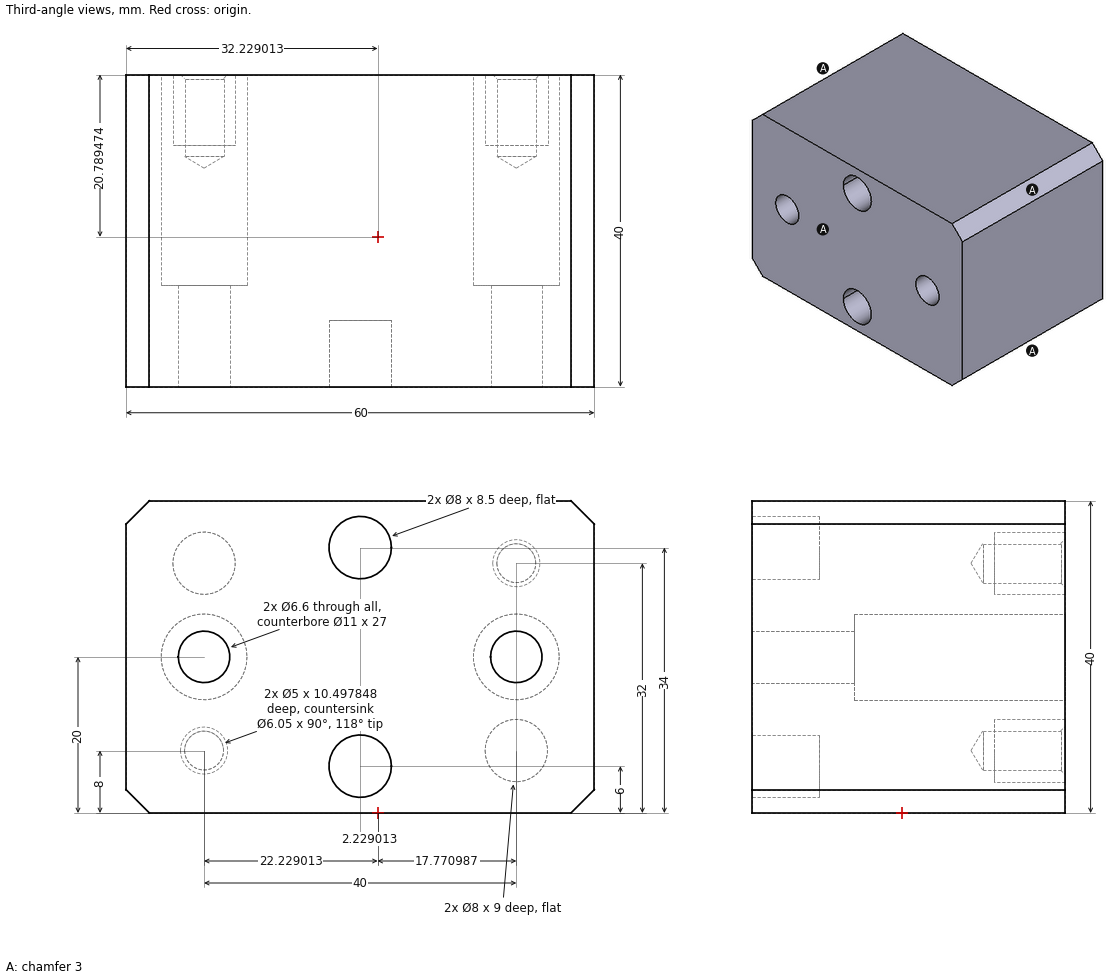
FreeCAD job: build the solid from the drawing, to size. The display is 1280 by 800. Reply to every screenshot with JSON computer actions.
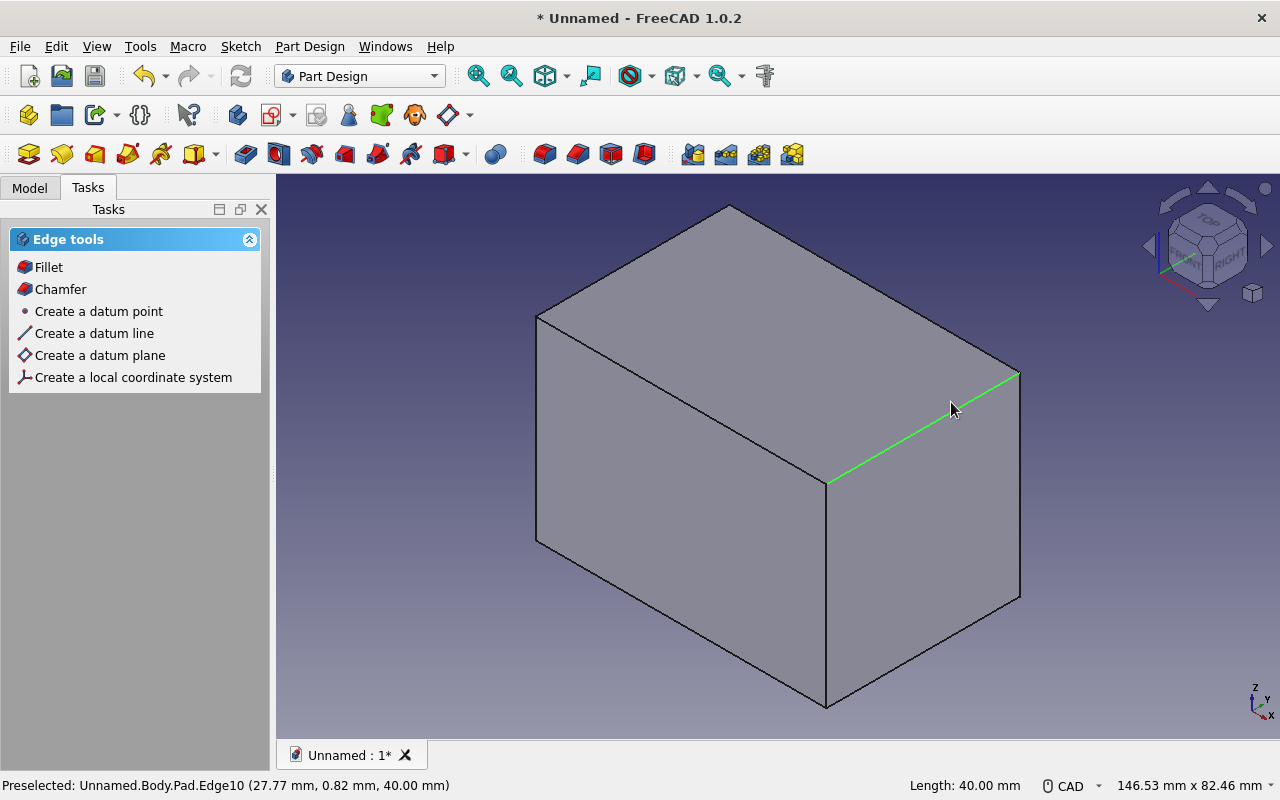
{"action": "key", "text": "2"}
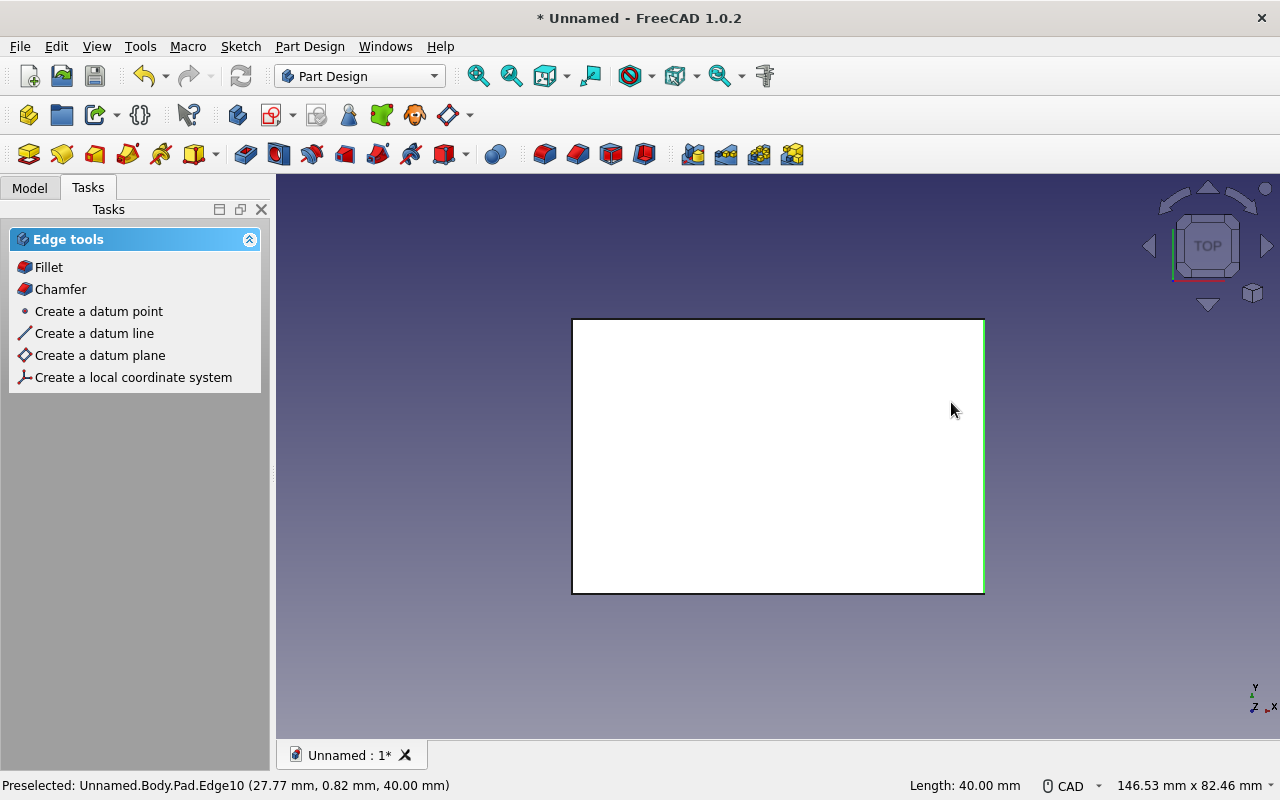
{"action": "left_click", "coordinate": [572, 456], "text": "ctrl"}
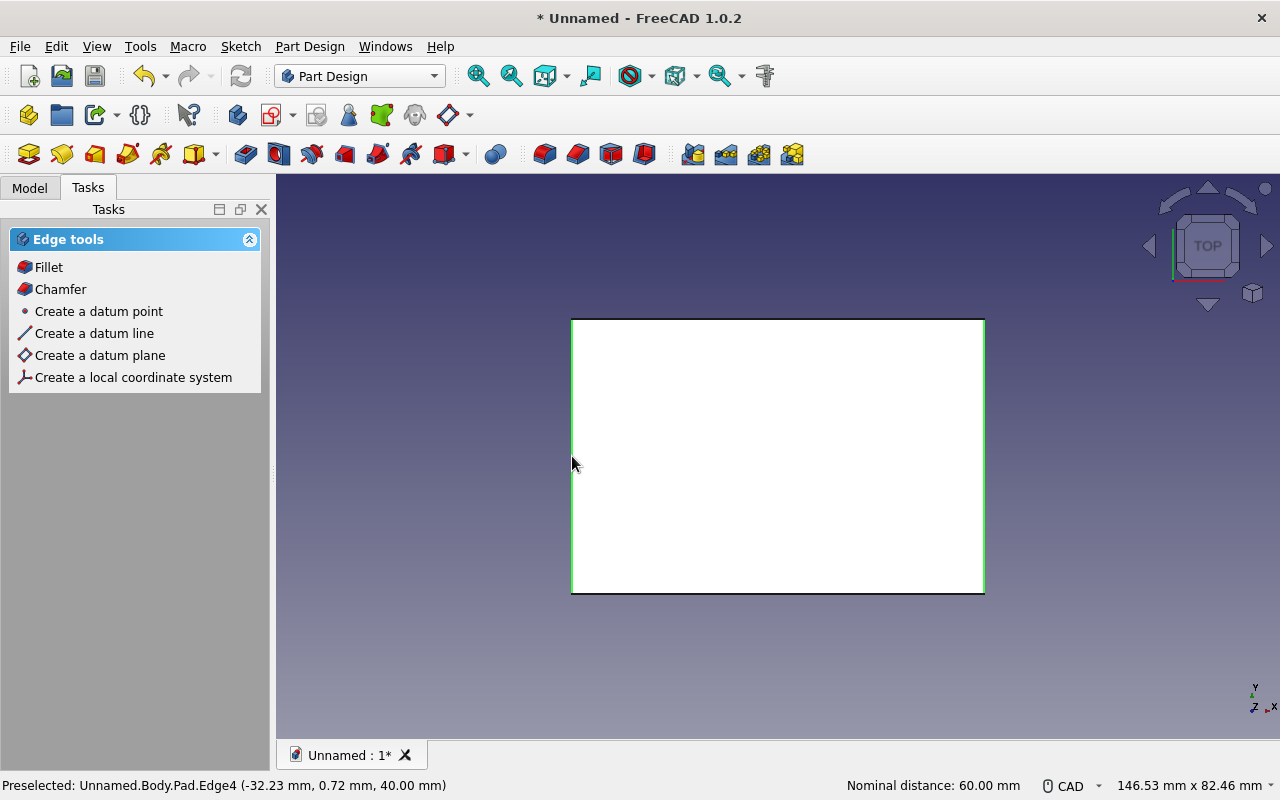
{"action": "key", "text": "1"}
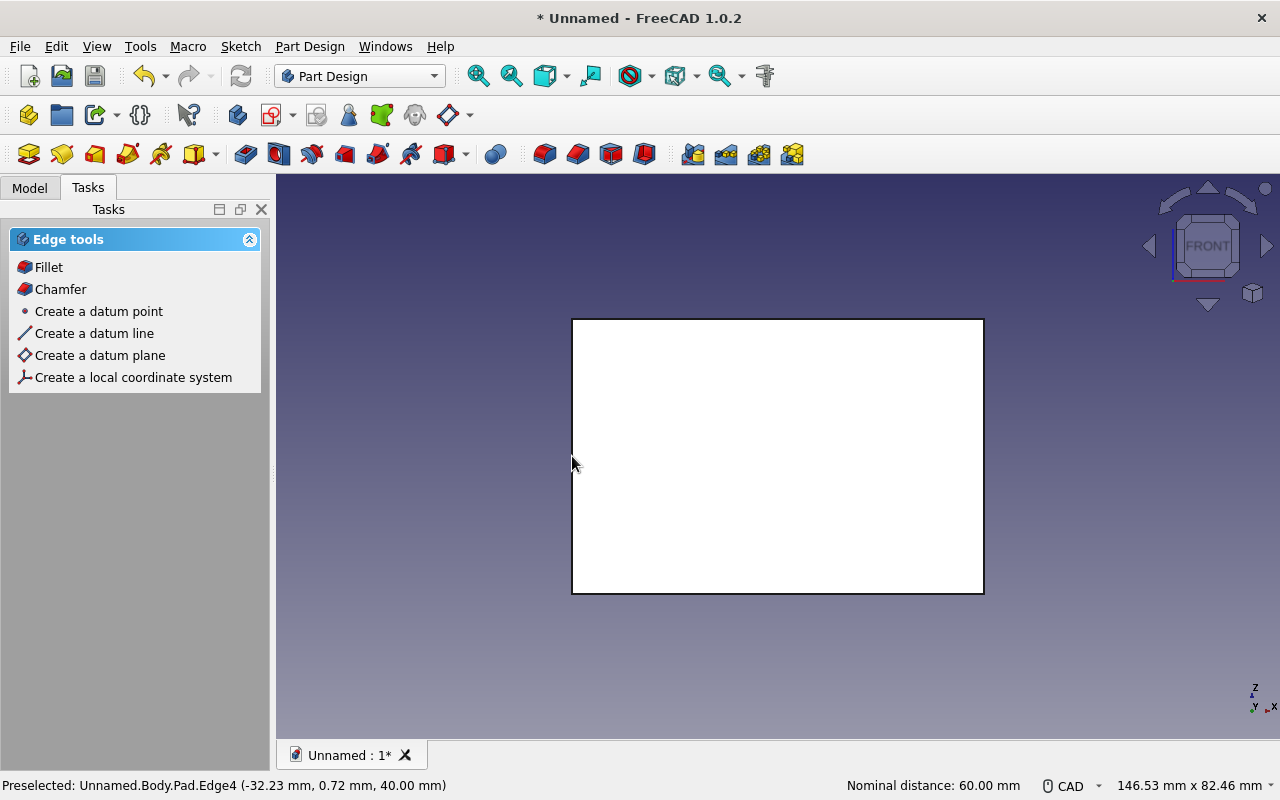
{"action": "key", "text": "3"}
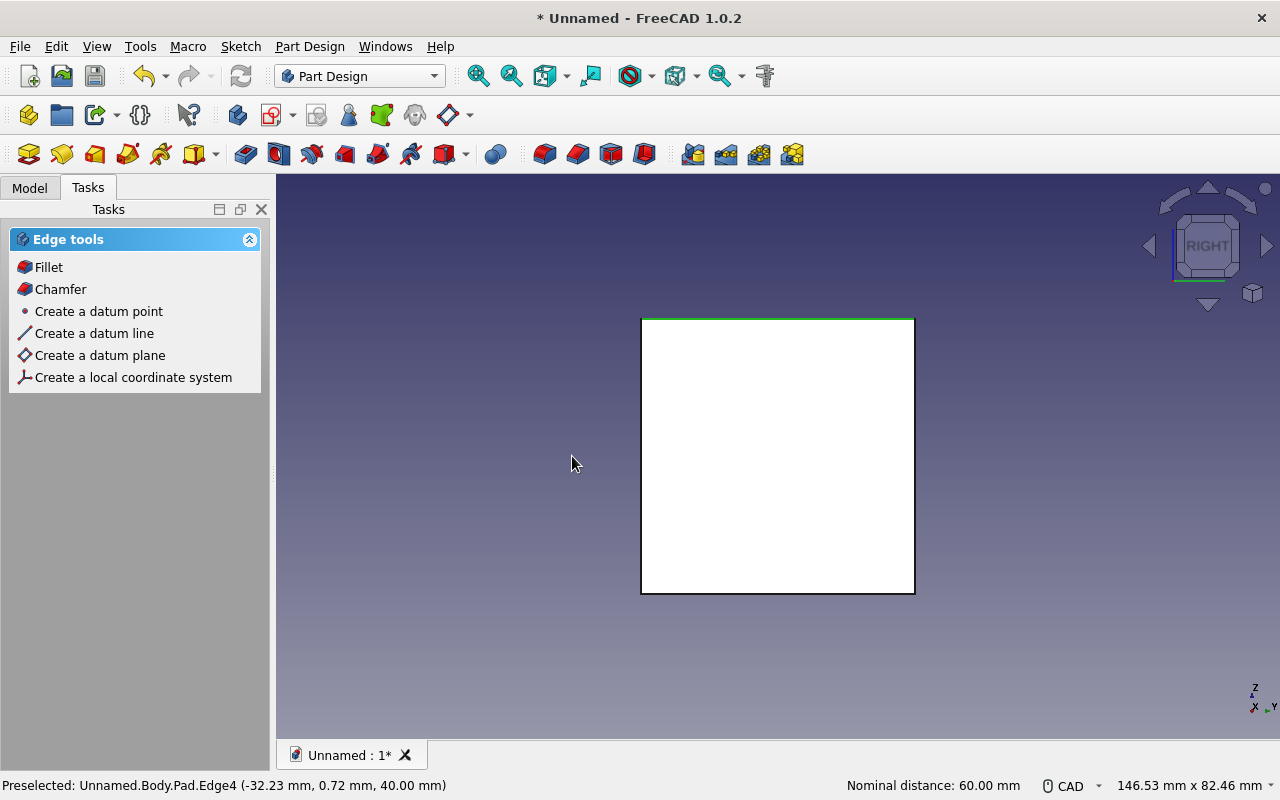
{"action": "left_click", "coordinate": [778, 593], "text": "ctrl"}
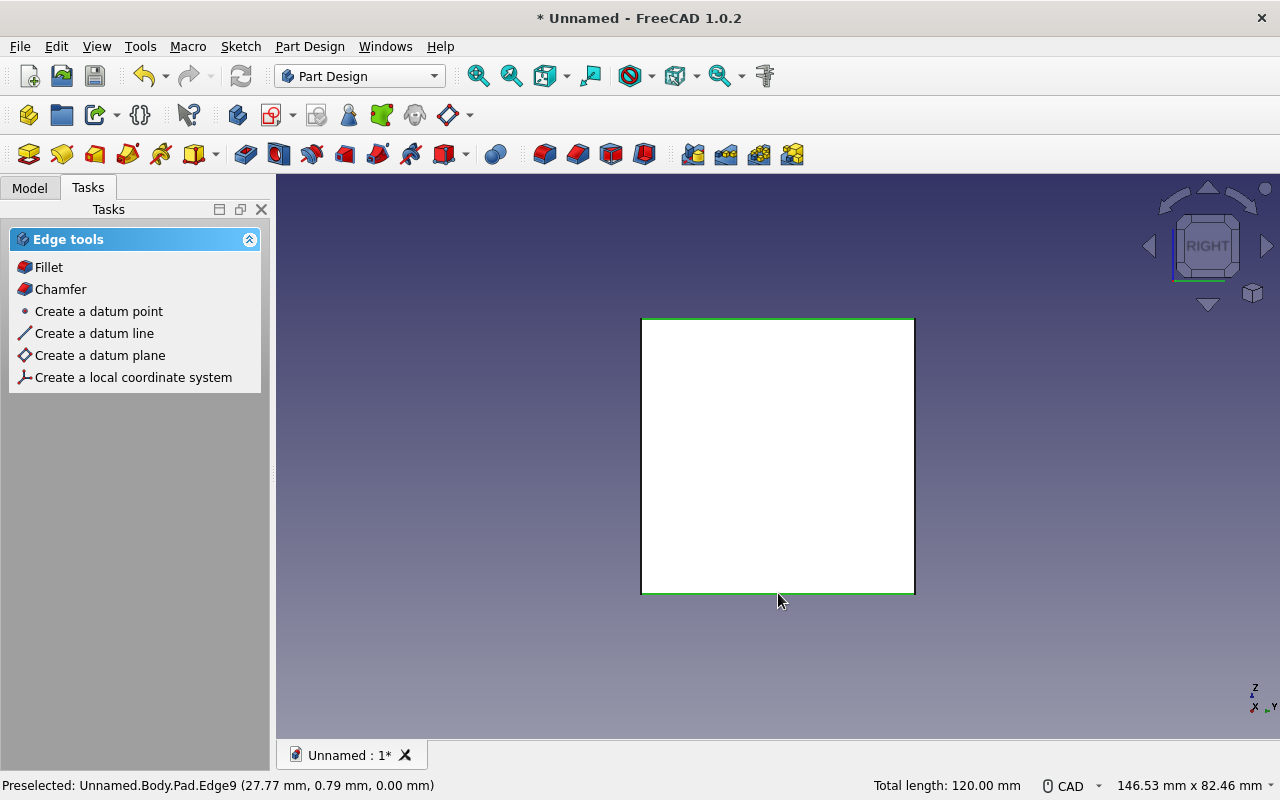
{"action": "key", "text": "5"}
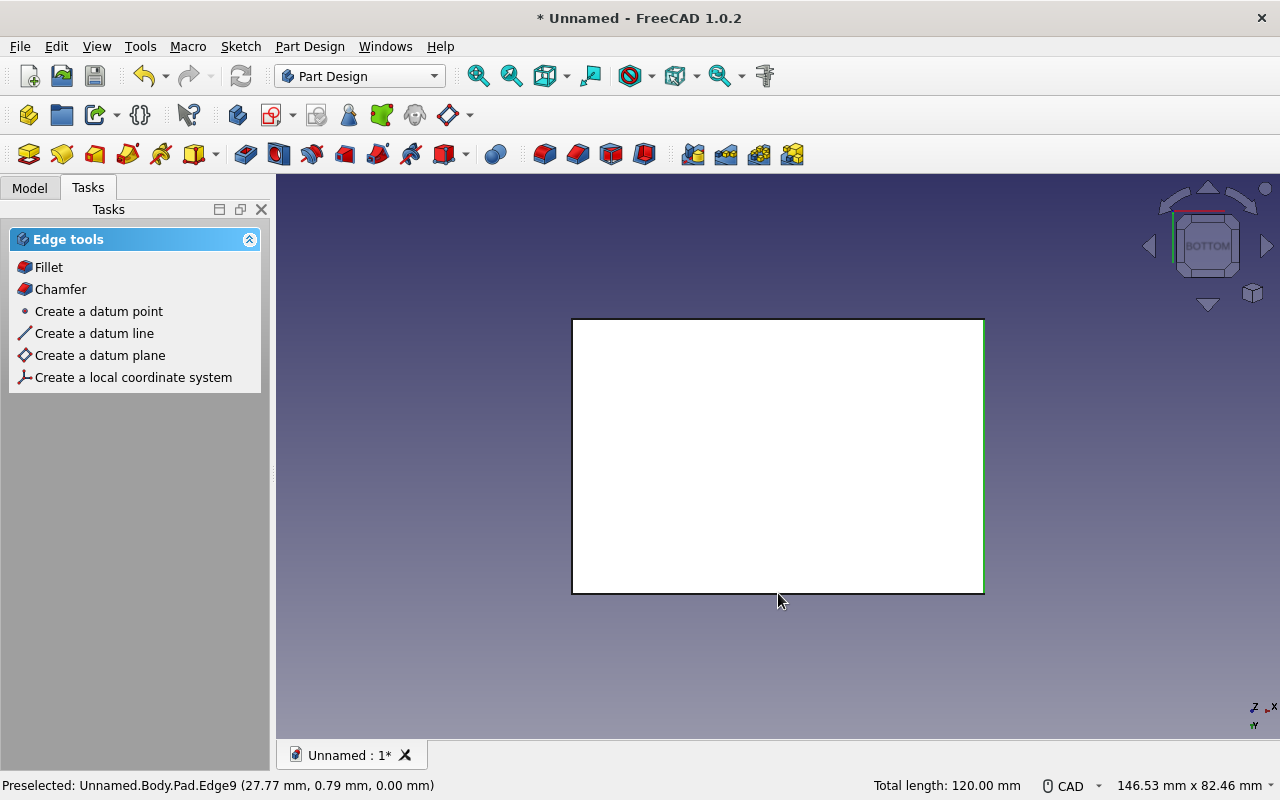
{"action": "left_click", "coordinate": [572, 455], "text": "ctrl"}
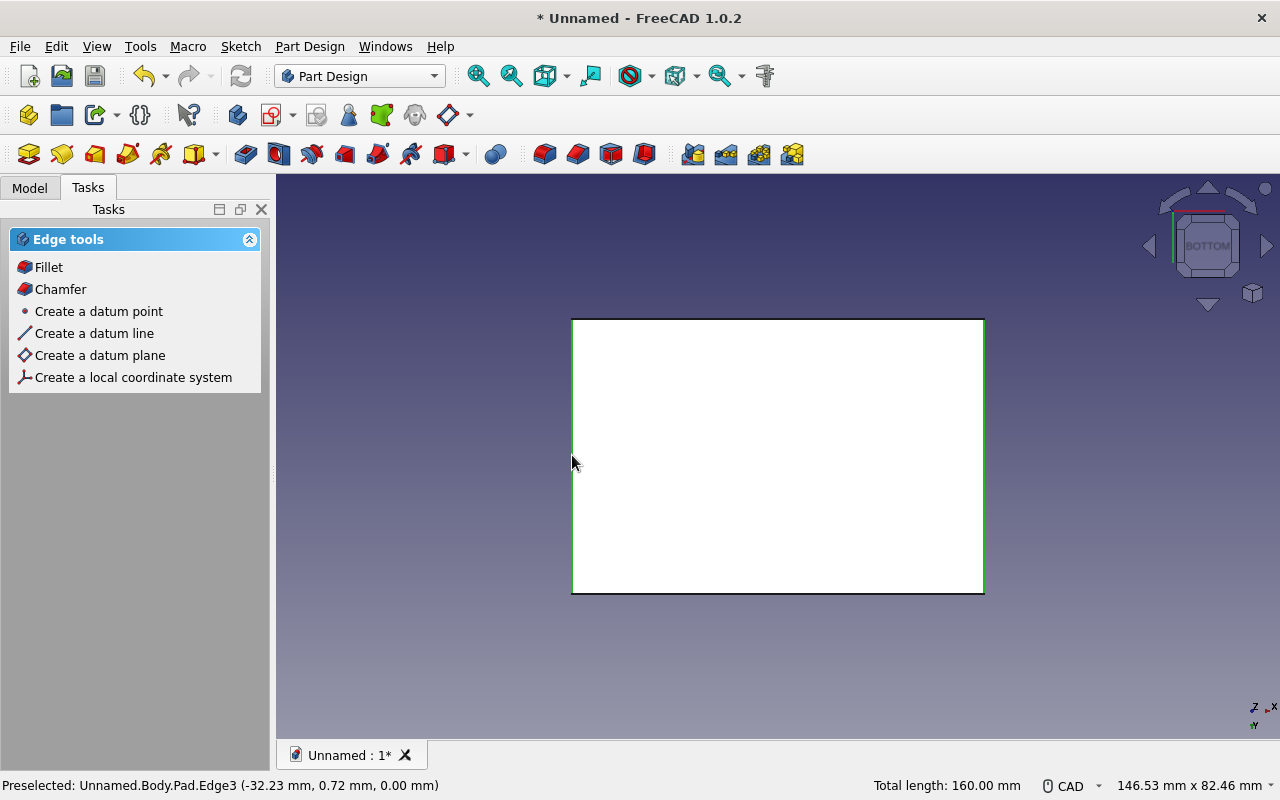
{"action": "left_click", "coordinate": [578, 154]}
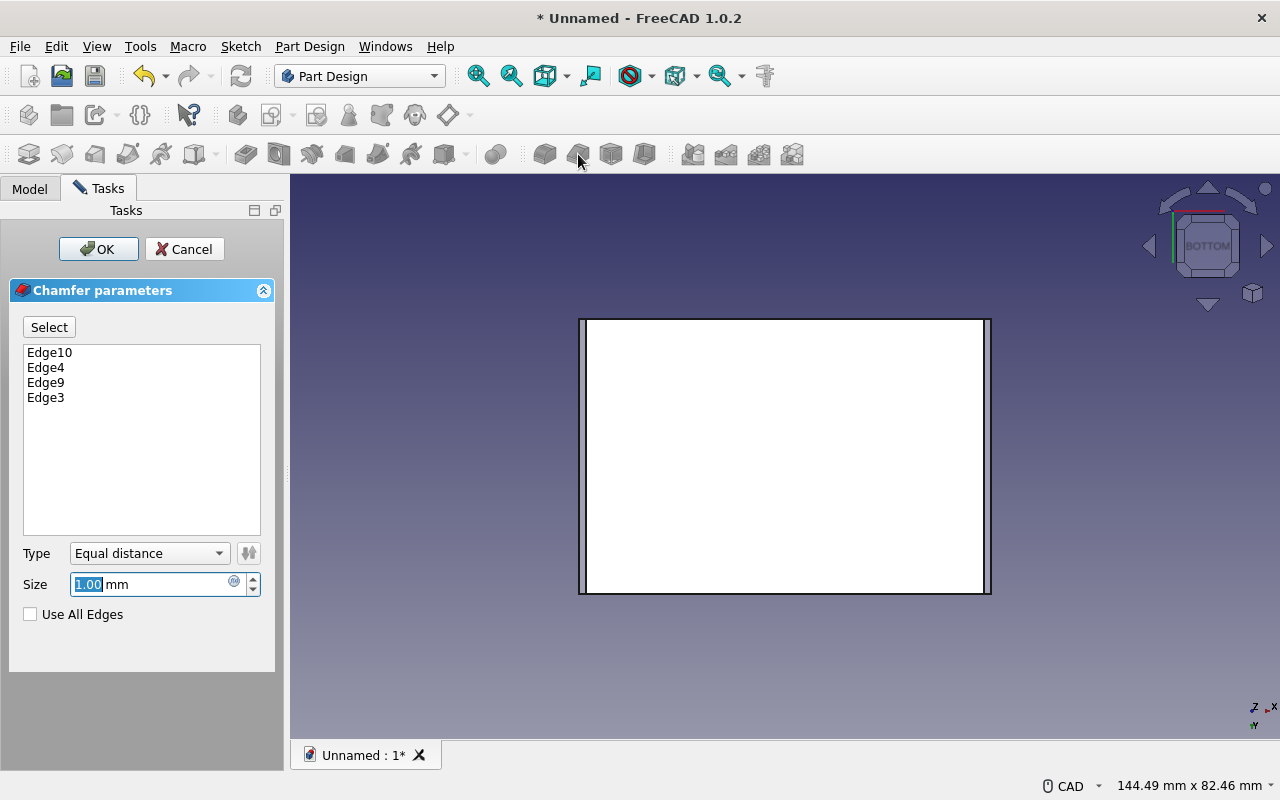
{"action": "type", "text": "3"}
{"action": "key", "text": "Tab"}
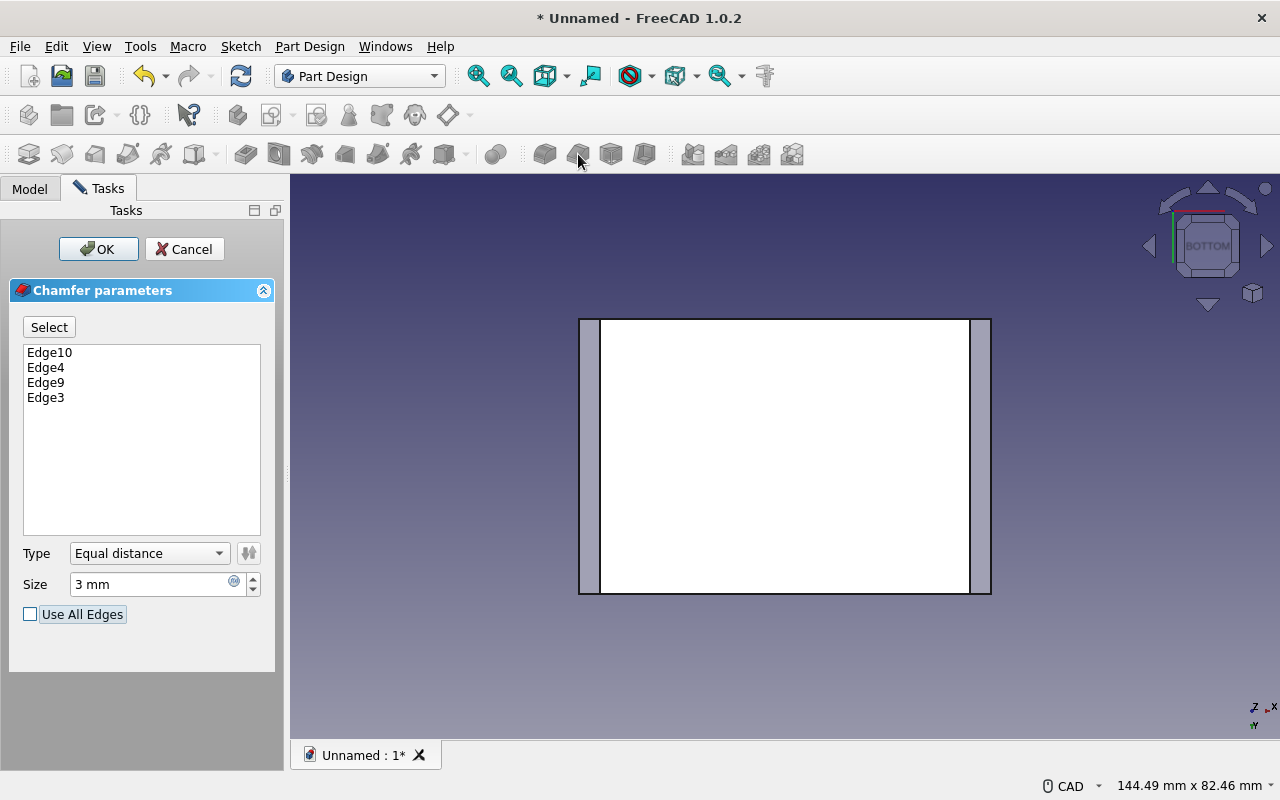
{"action": "left_click", "coordinate": [99, 249]}